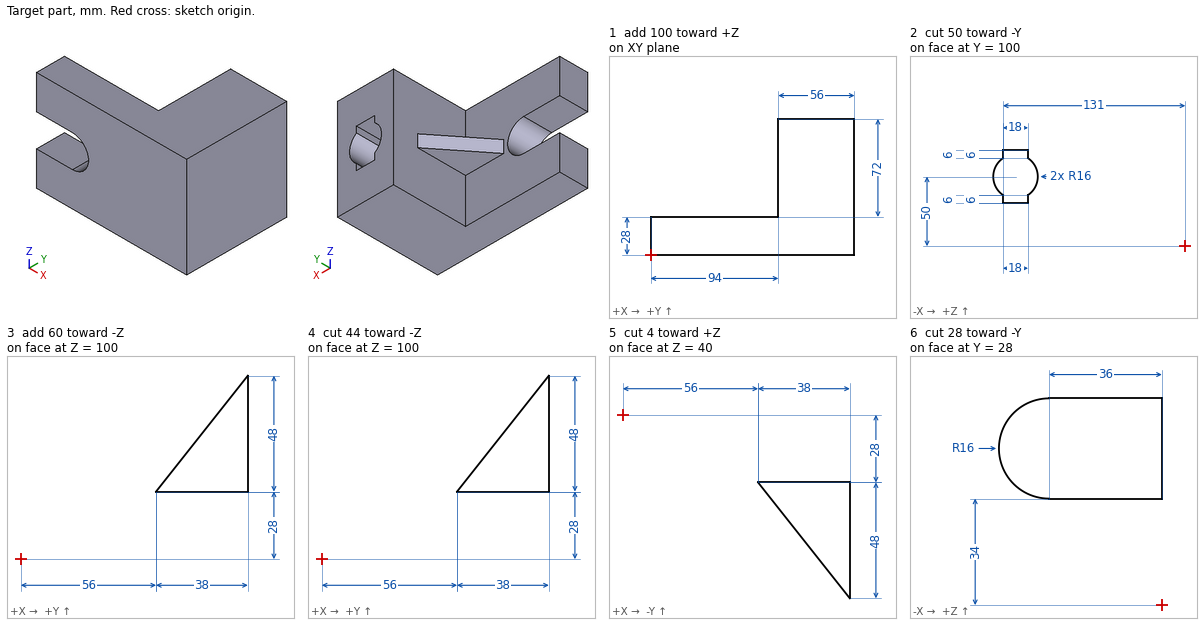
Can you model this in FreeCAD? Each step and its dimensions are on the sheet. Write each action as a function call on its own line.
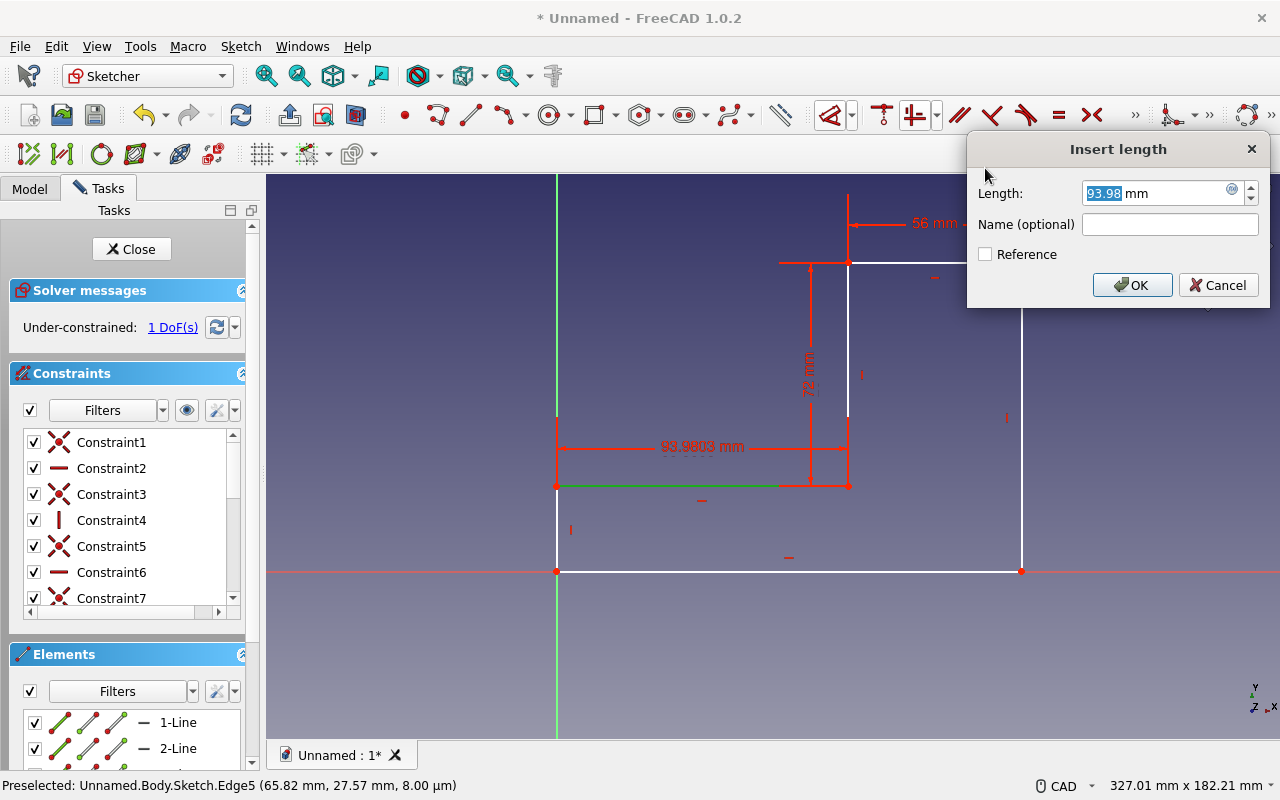
text(94)
key(Return)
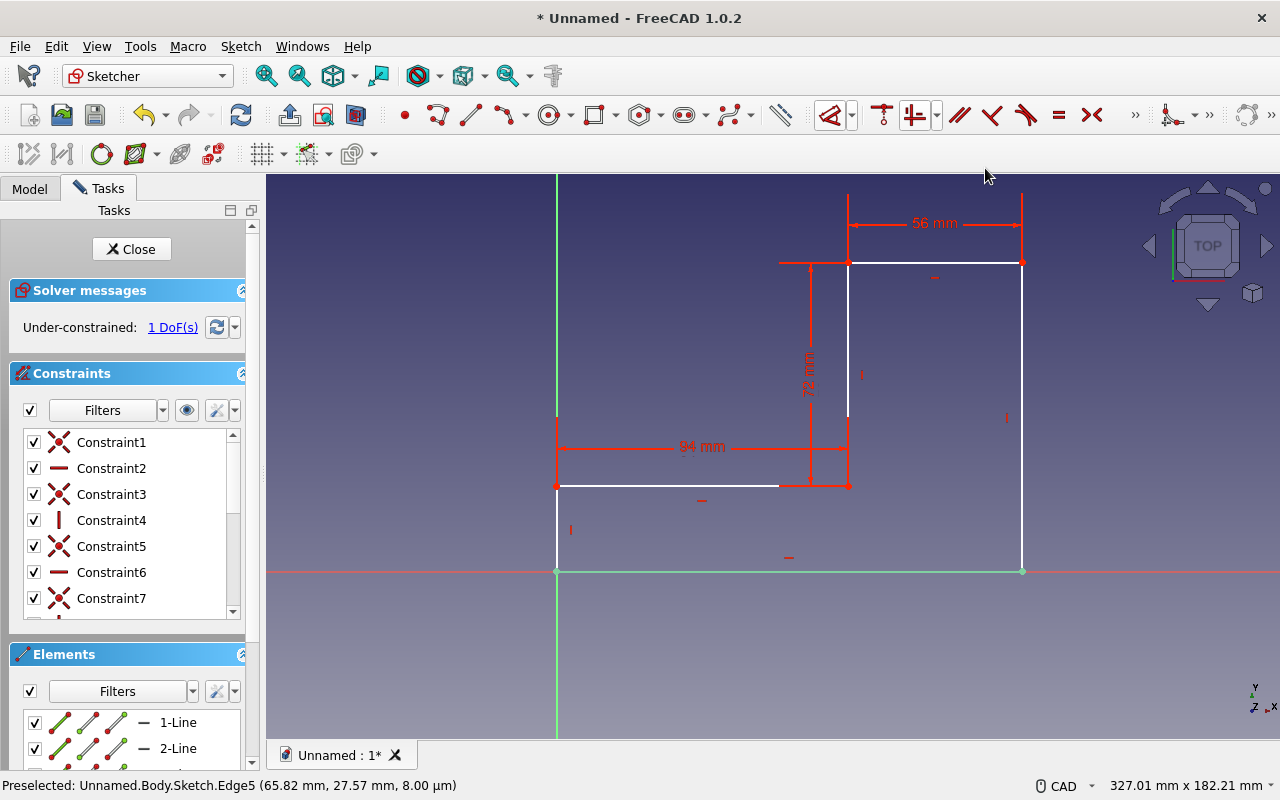
click(557, 512)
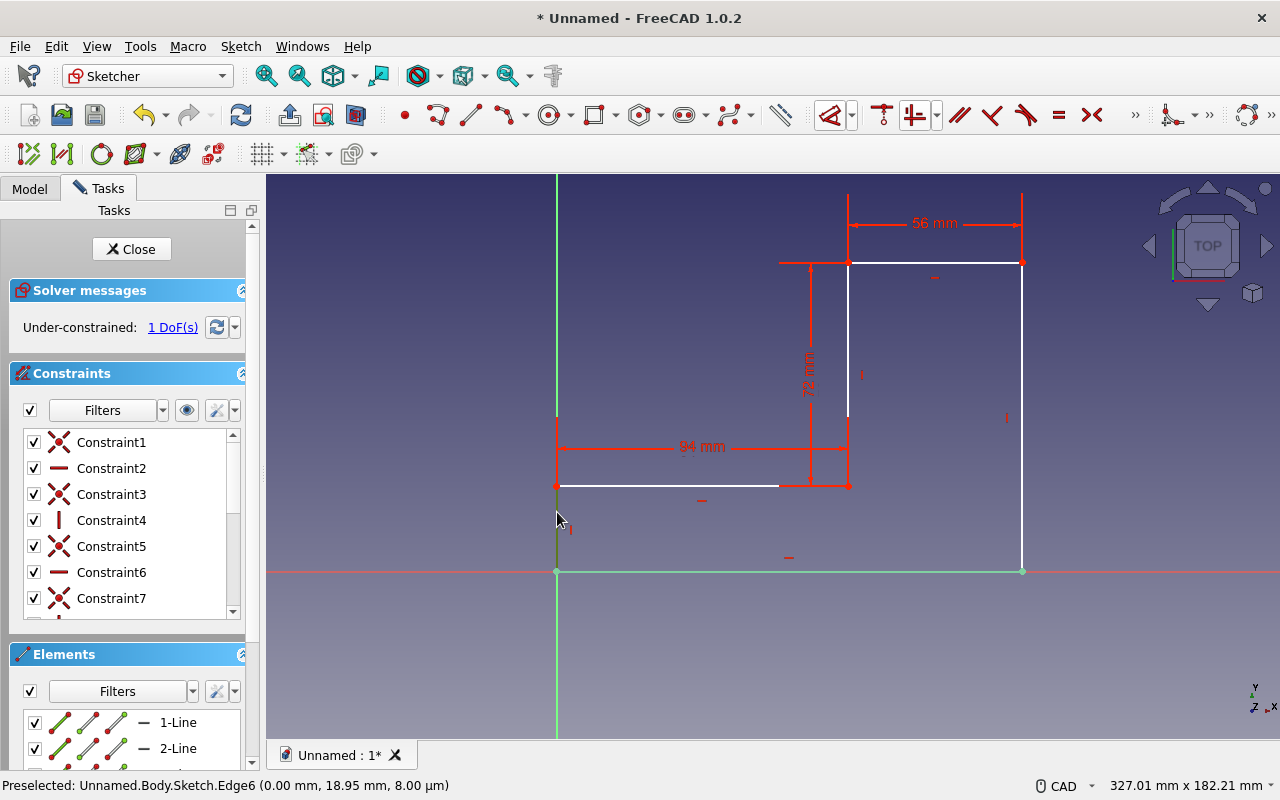
key(i)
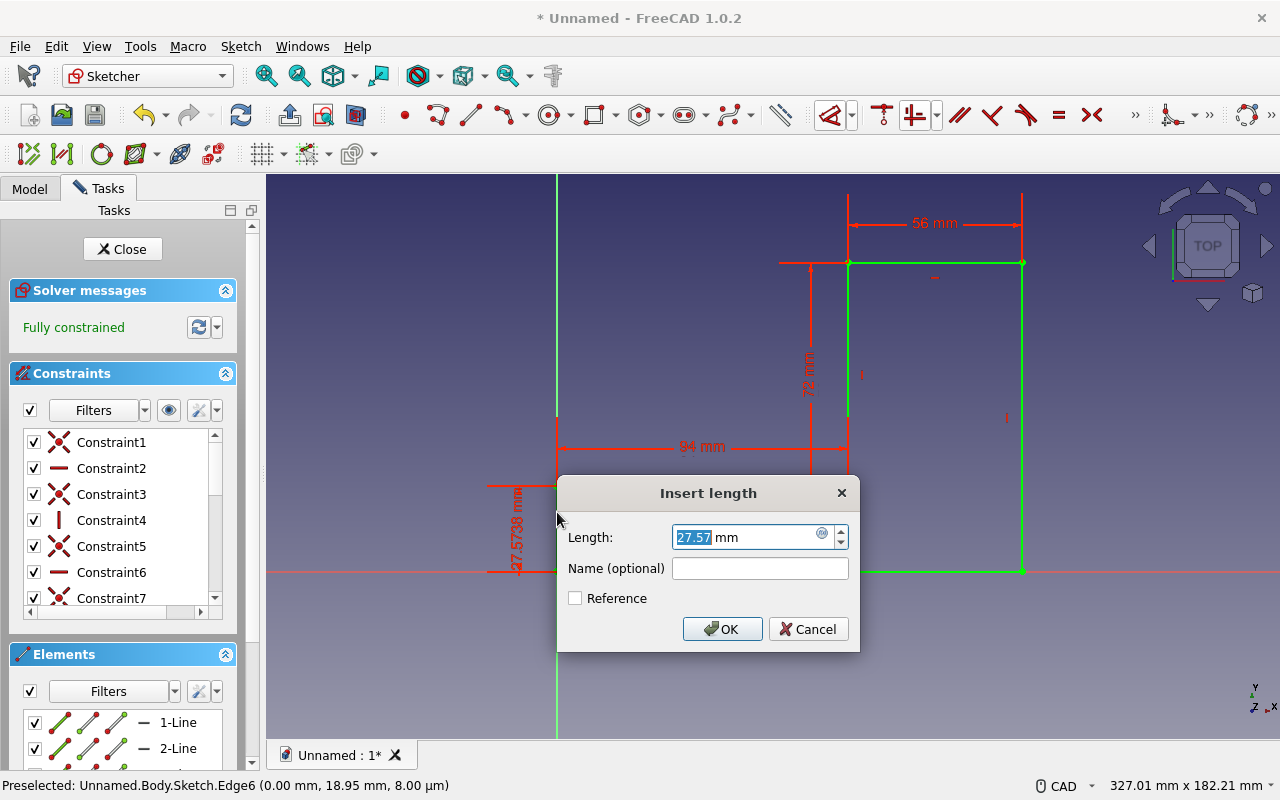
text(28)
key(Return)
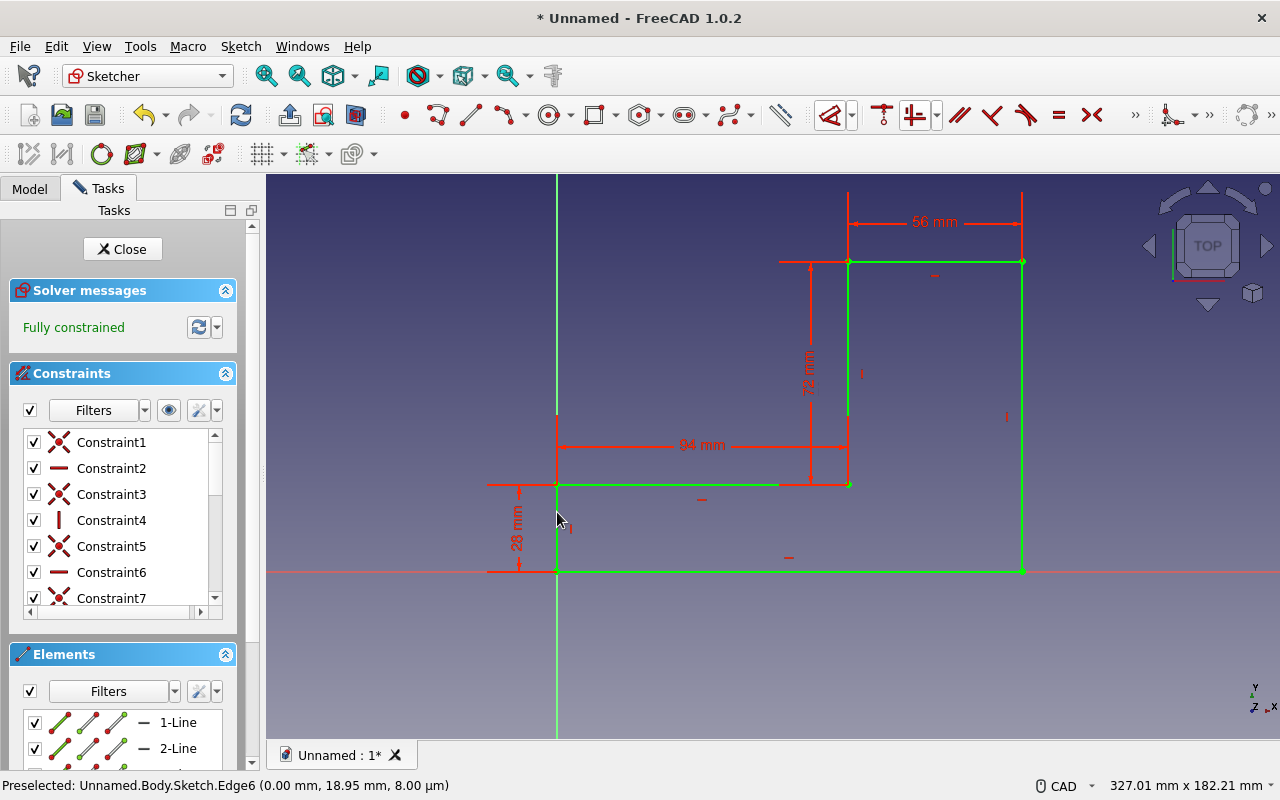
click(123, 249)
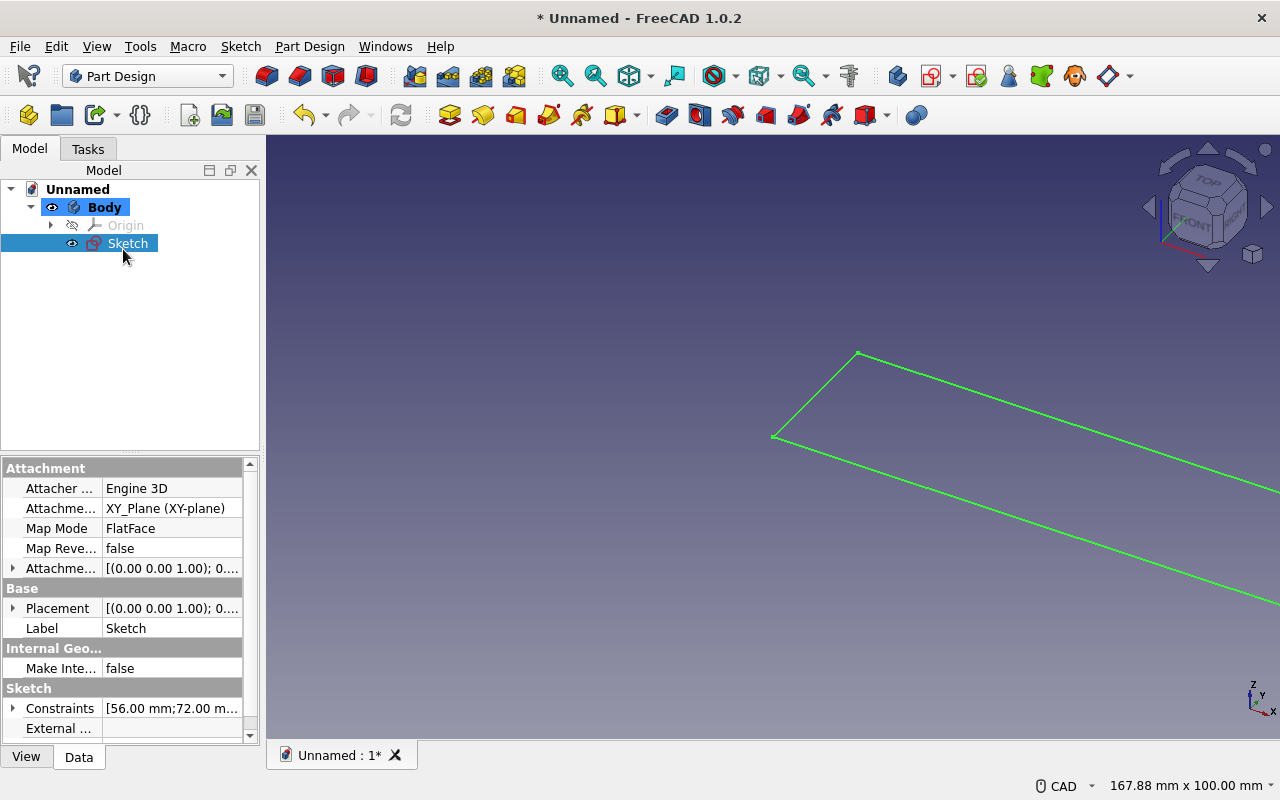
click(450, 116)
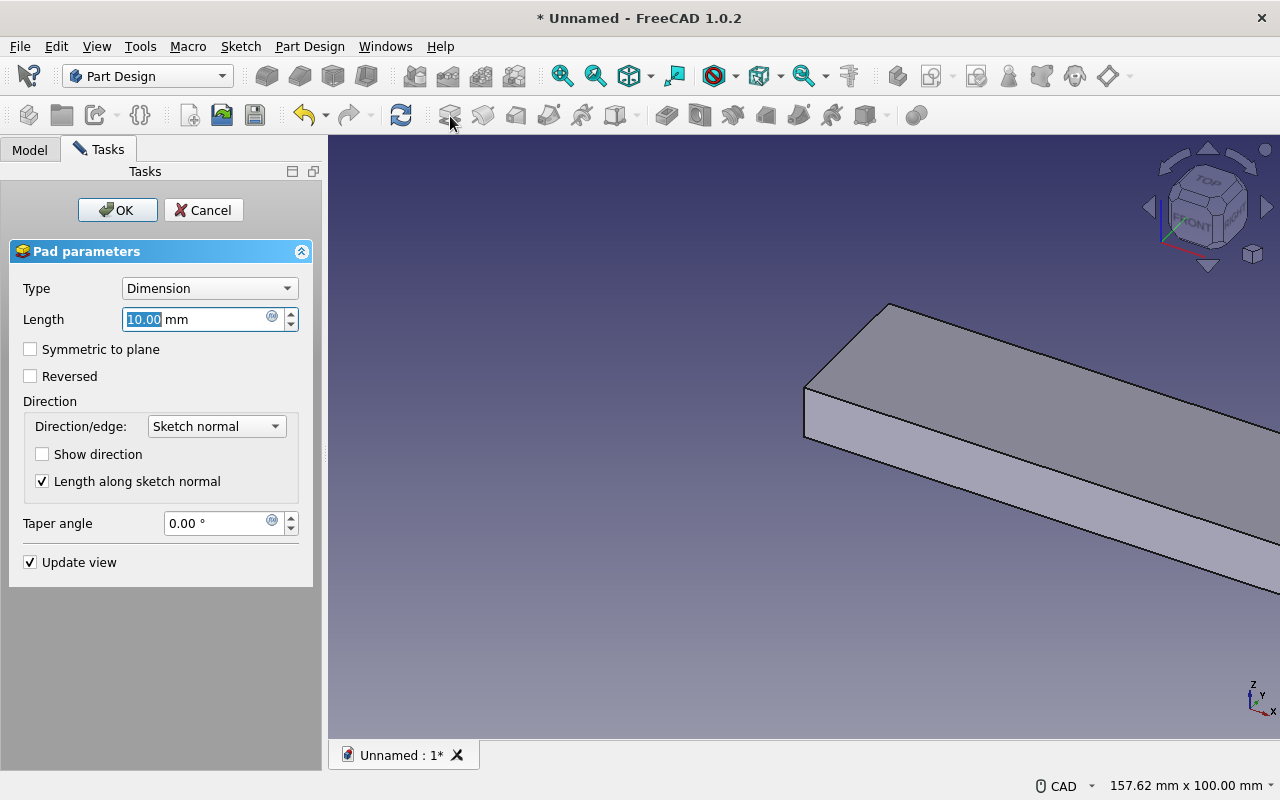
text(100)
key(Tab)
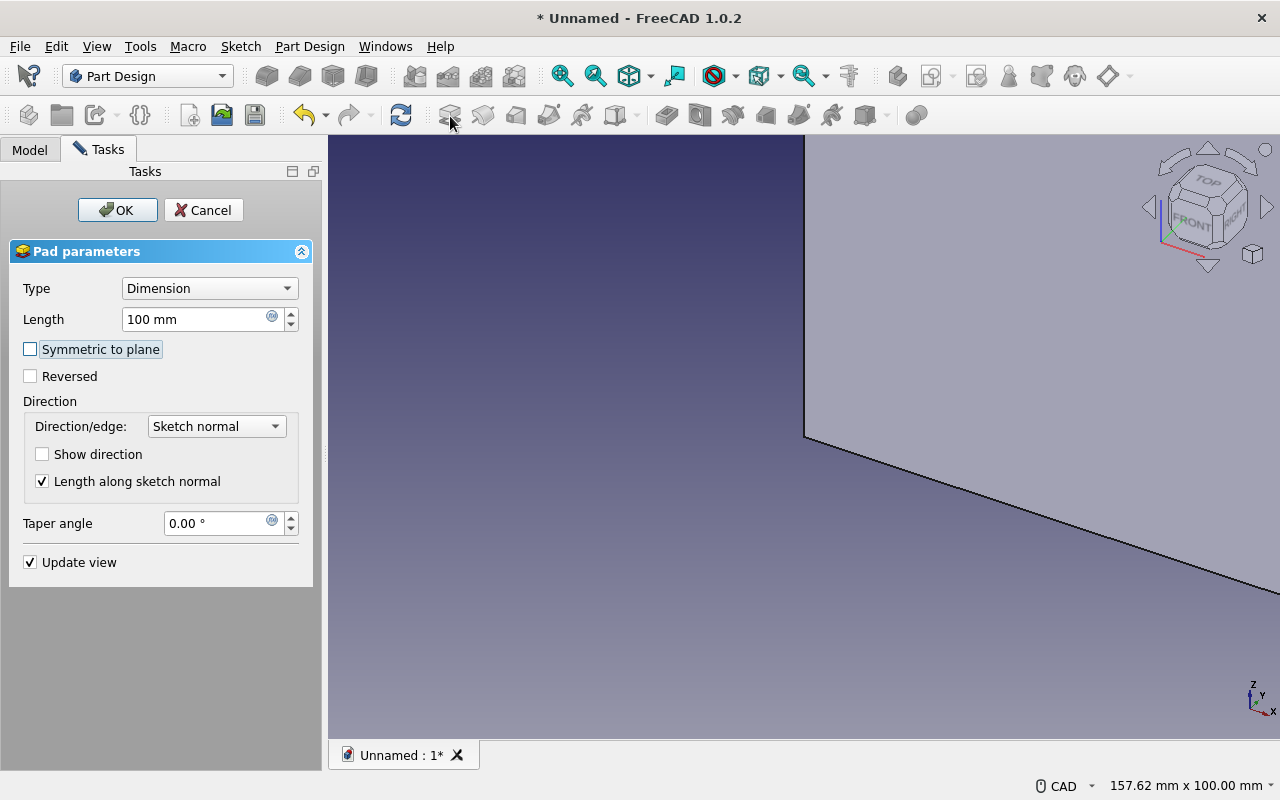
click(118, 210)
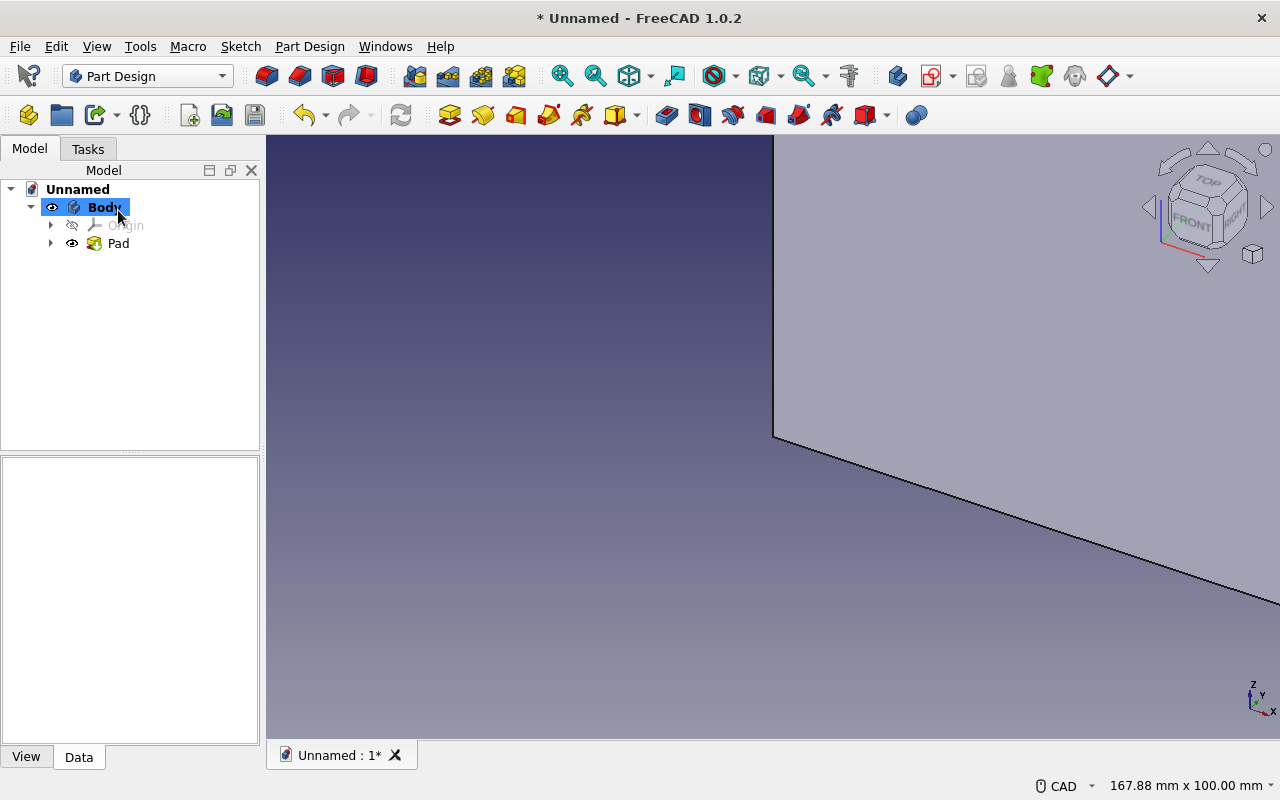
click(563, 76)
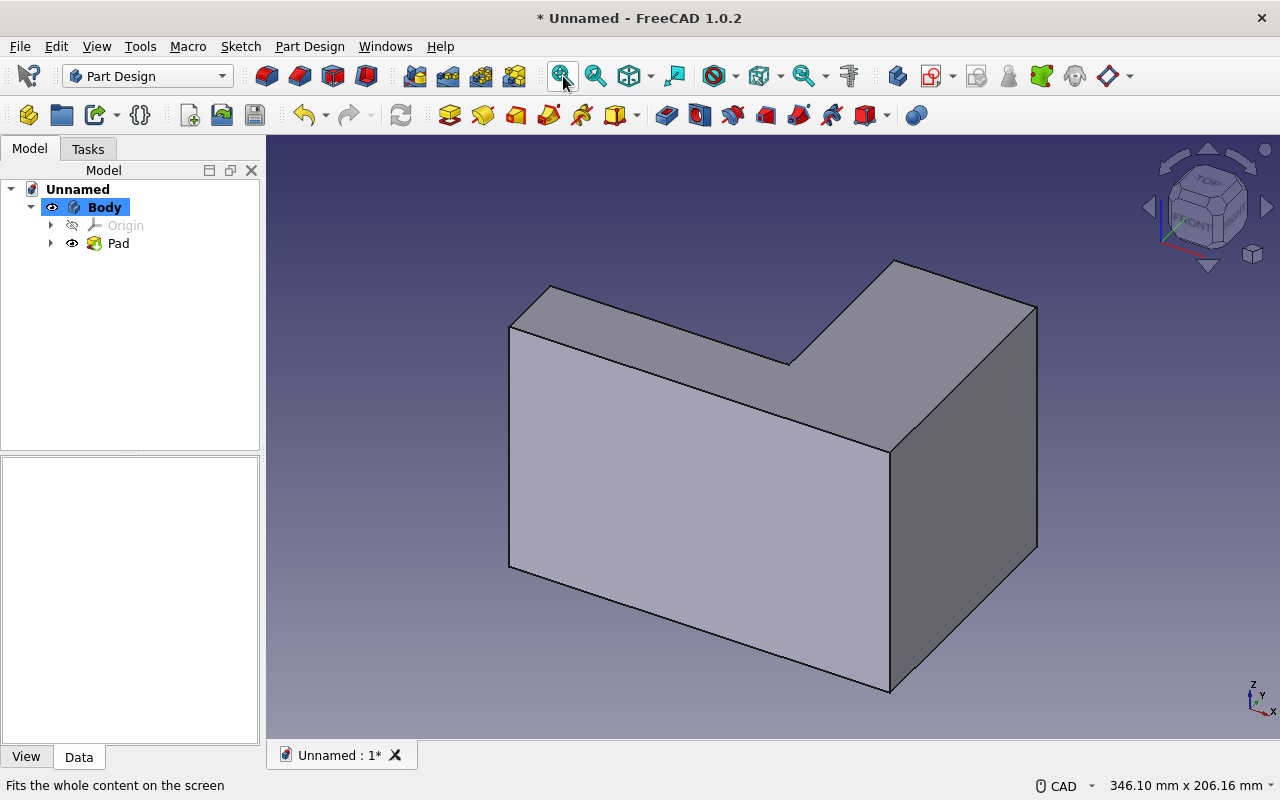
key(4)